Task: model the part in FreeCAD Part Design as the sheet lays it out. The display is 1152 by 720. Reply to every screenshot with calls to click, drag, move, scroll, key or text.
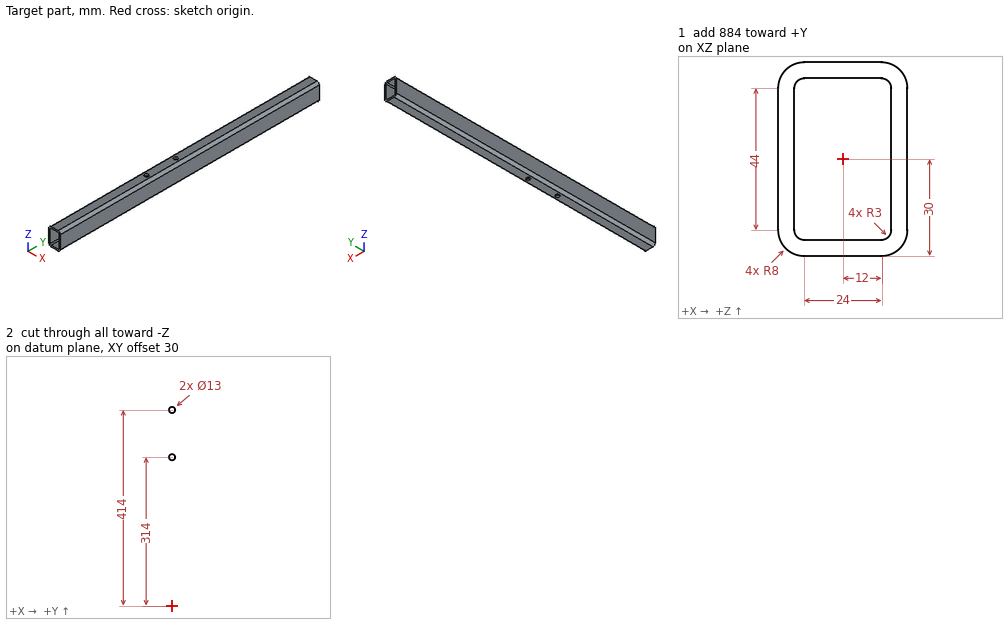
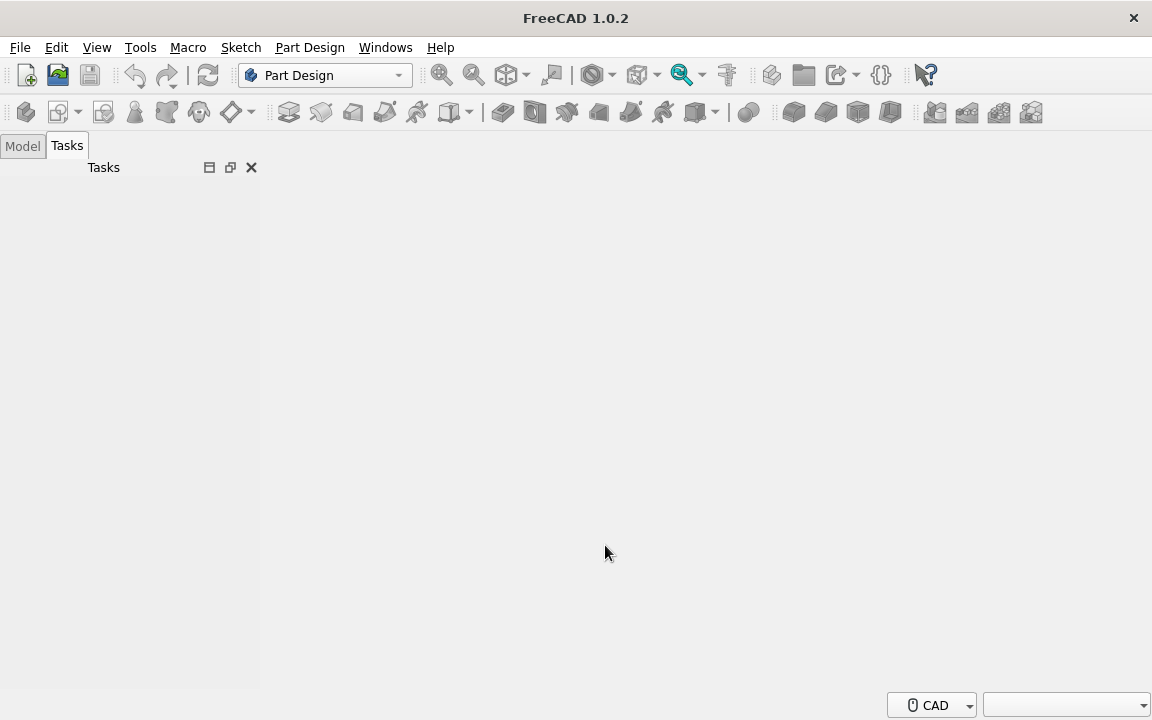
key(ctrl+n)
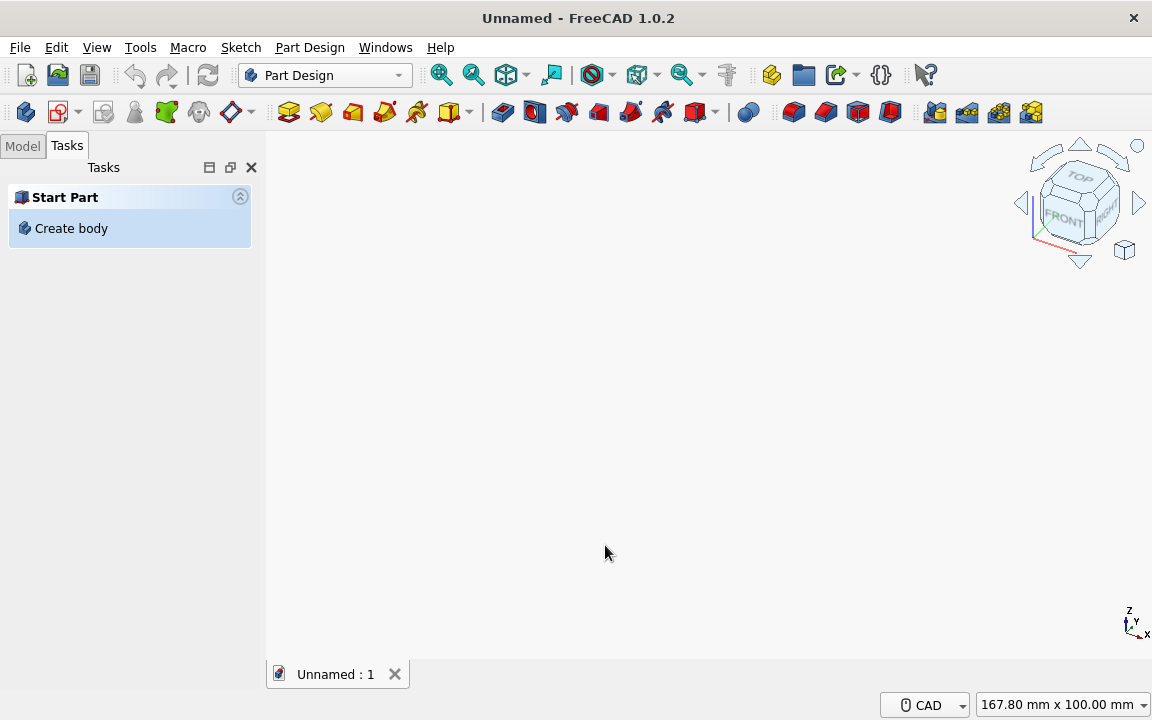
click(58, 112)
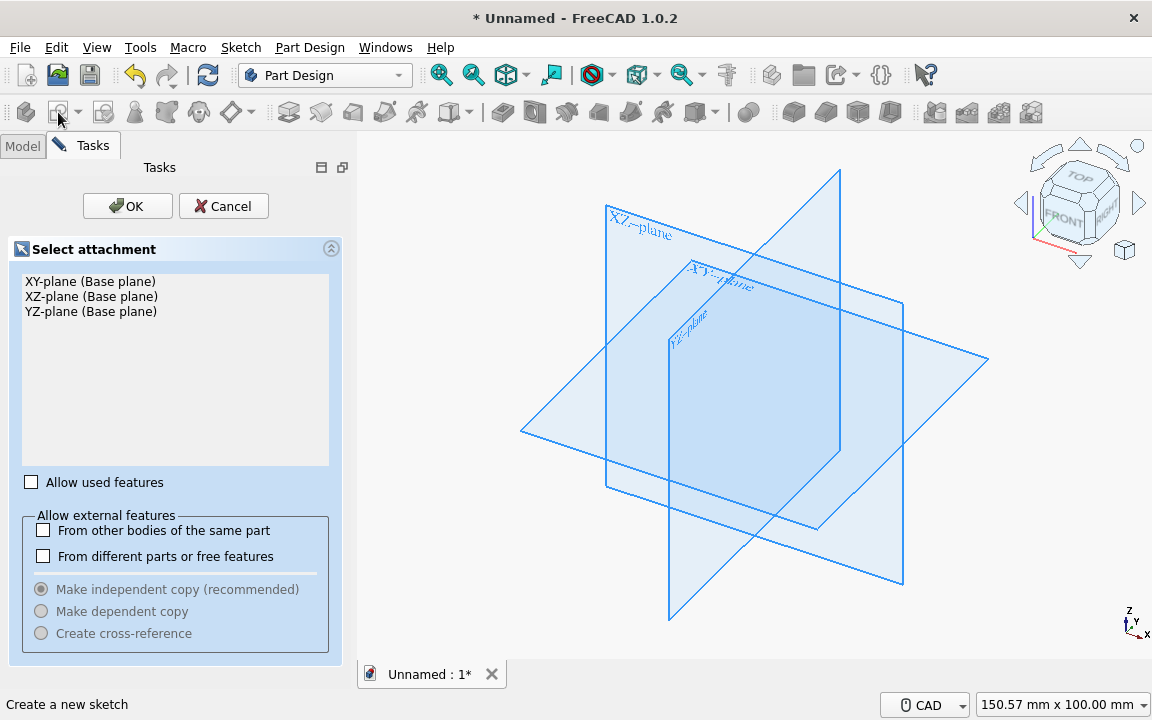
click(82, 296)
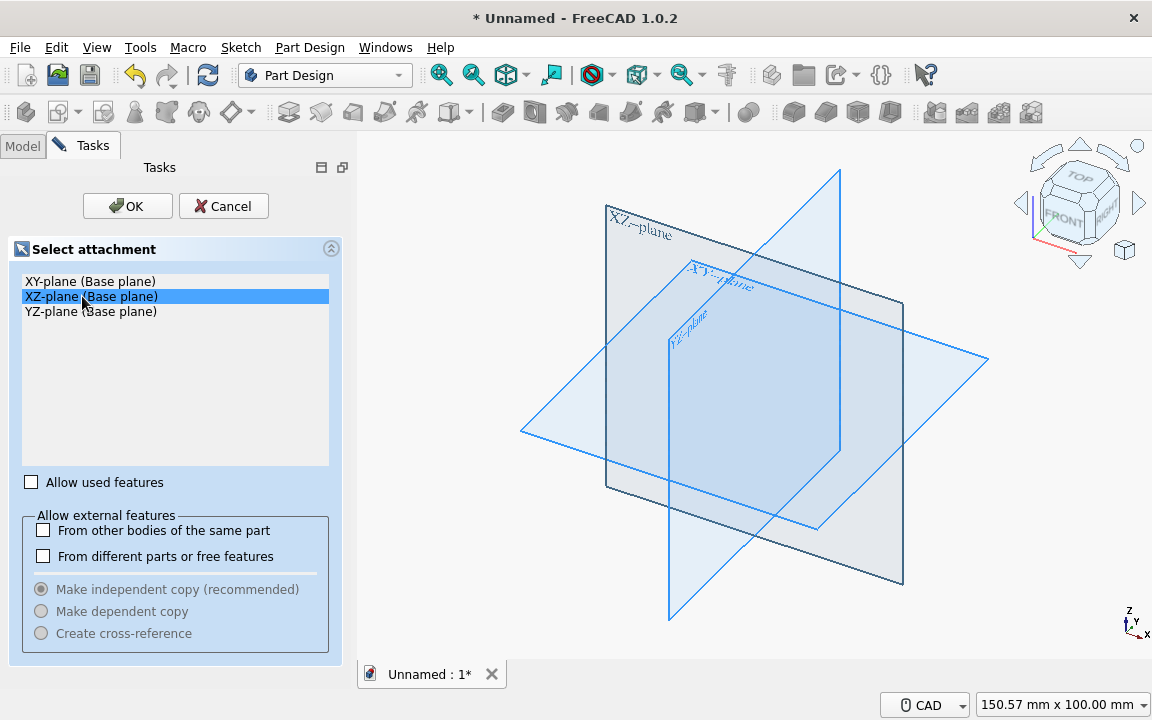
click(128, 206)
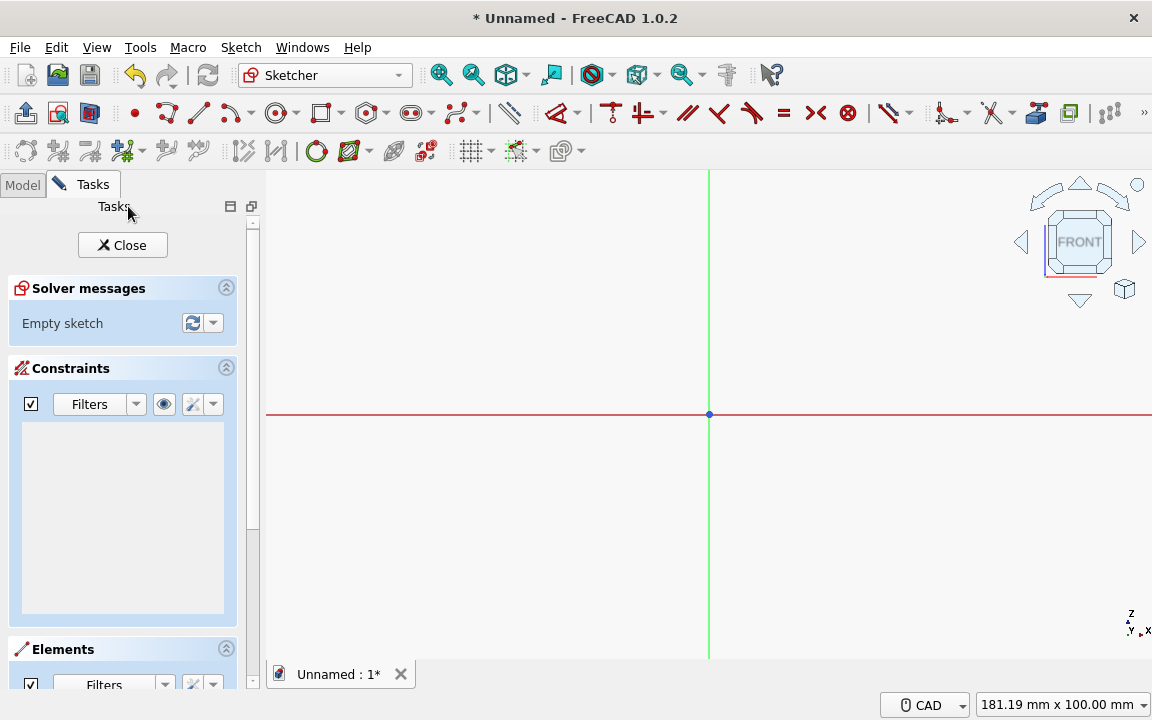
key(g)
key(l)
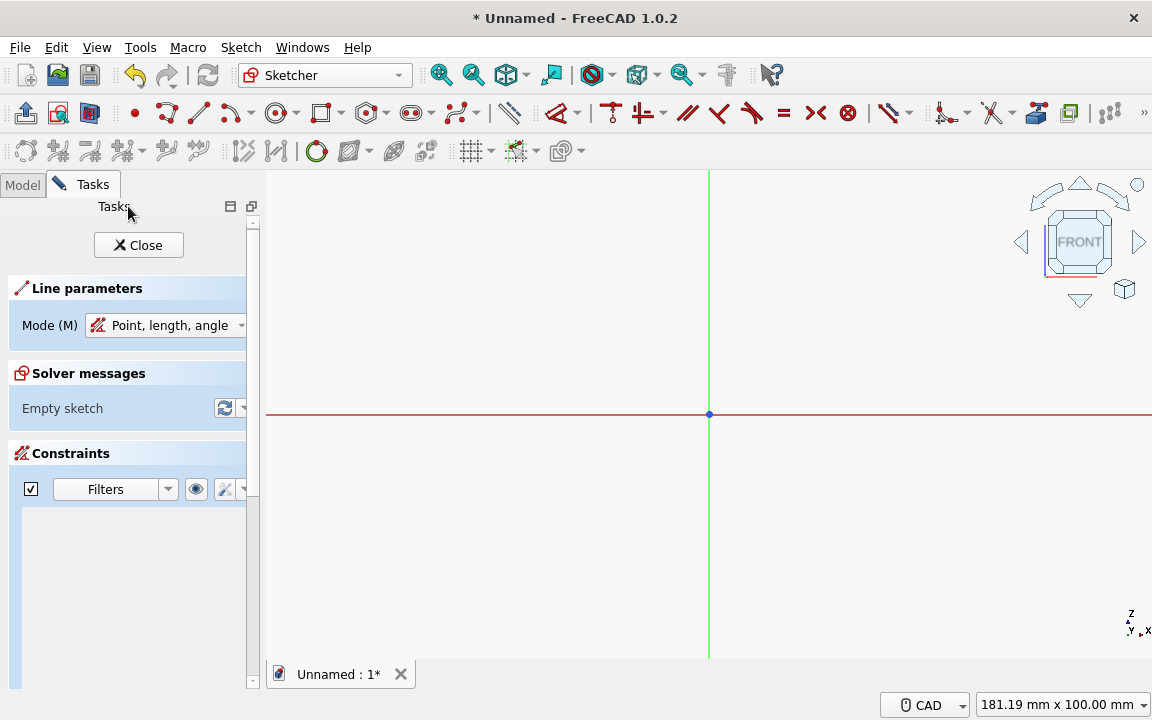
click(768, 561)
click(650, 561)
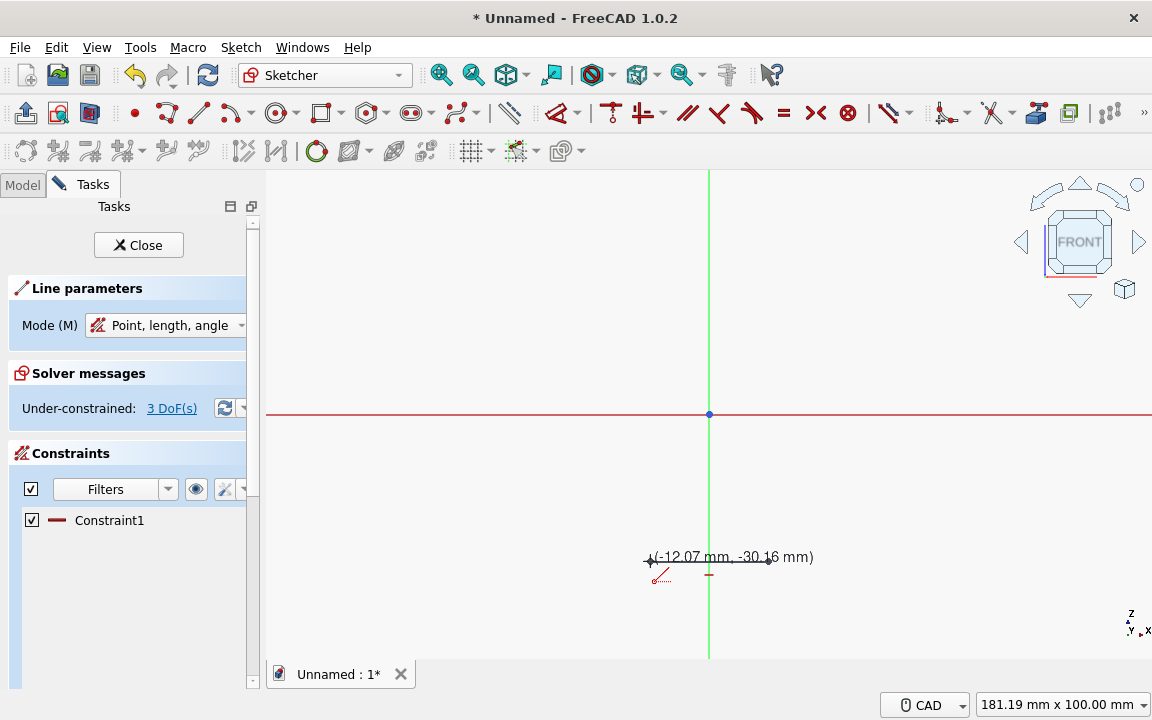
click(611, 522)
click(611, 307)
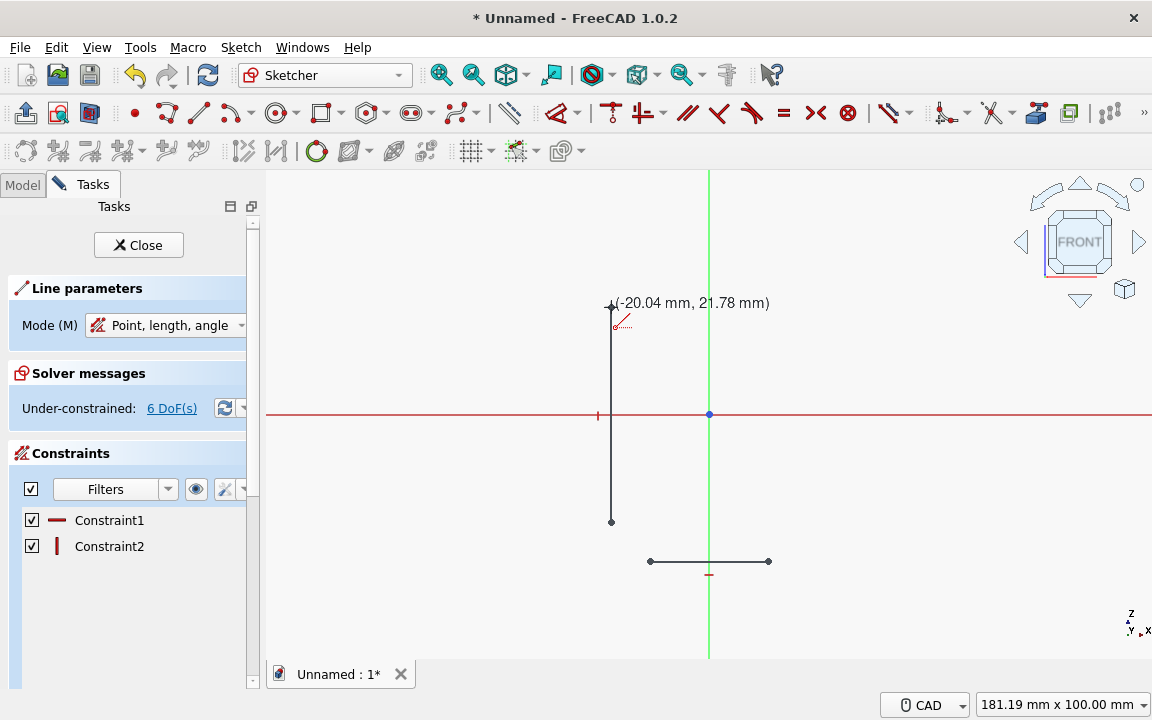
click(650, 268)
click(768, 268)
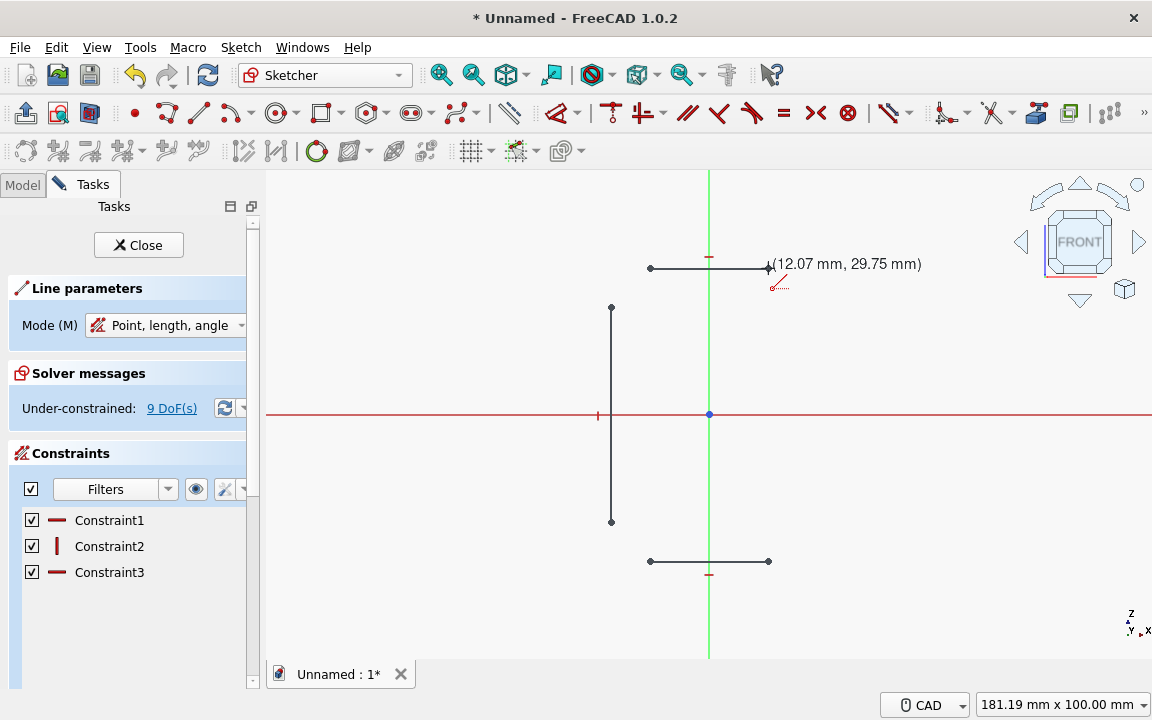
click(807, 307)
click(807, 522)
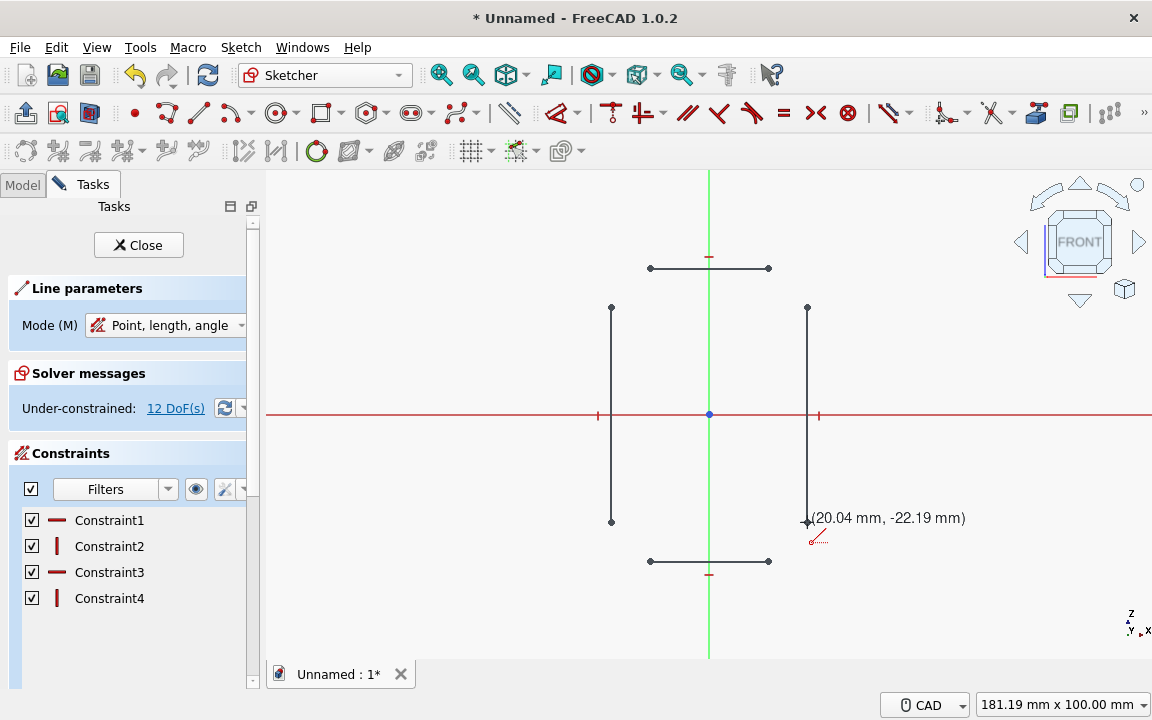
key(g)
key(3)
key(a)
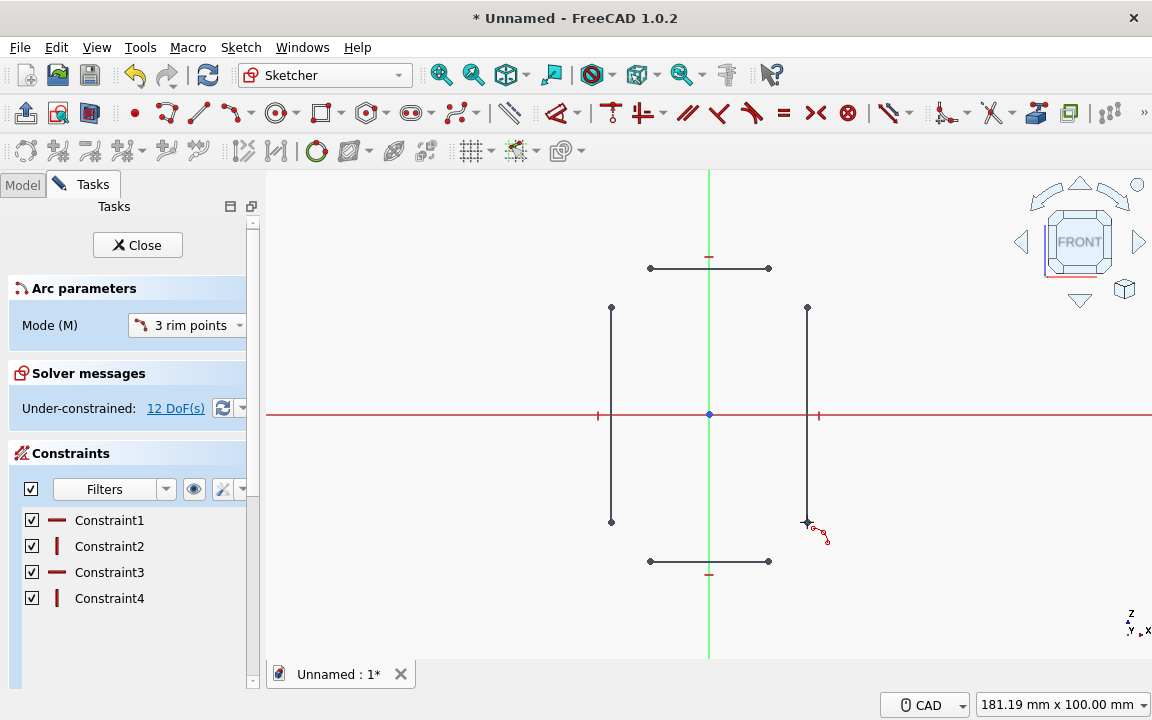
click(650, 562)
click(611, 523)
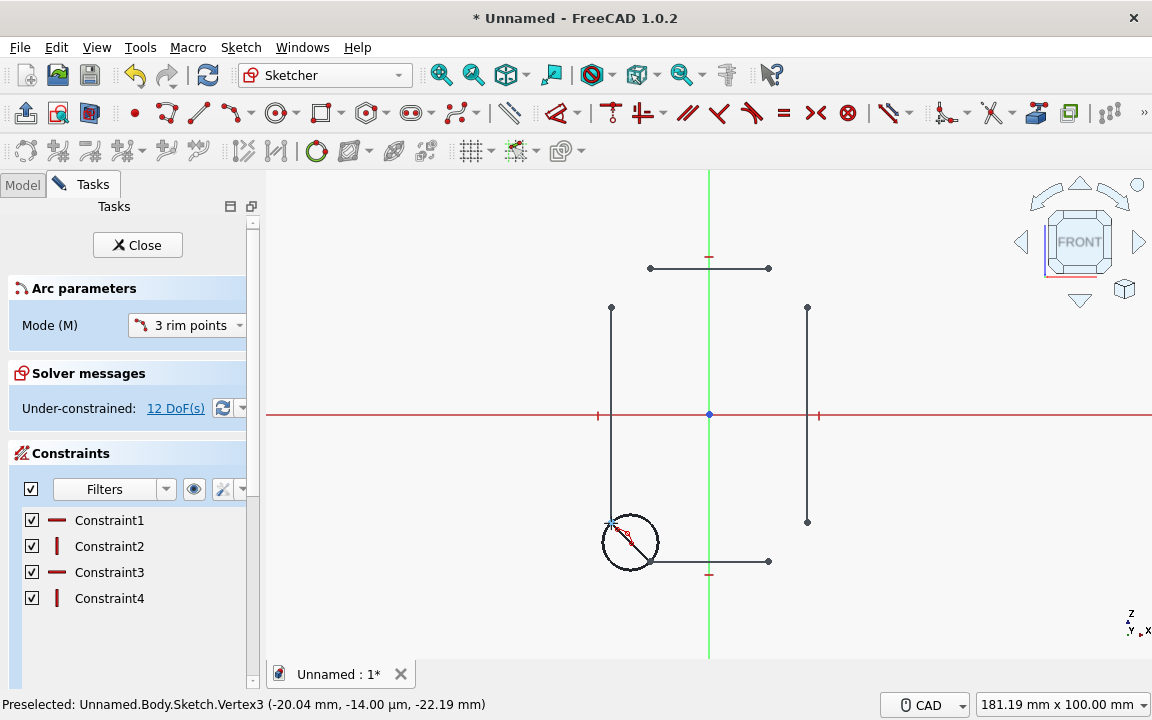
scroll(623, 550, up, 2)